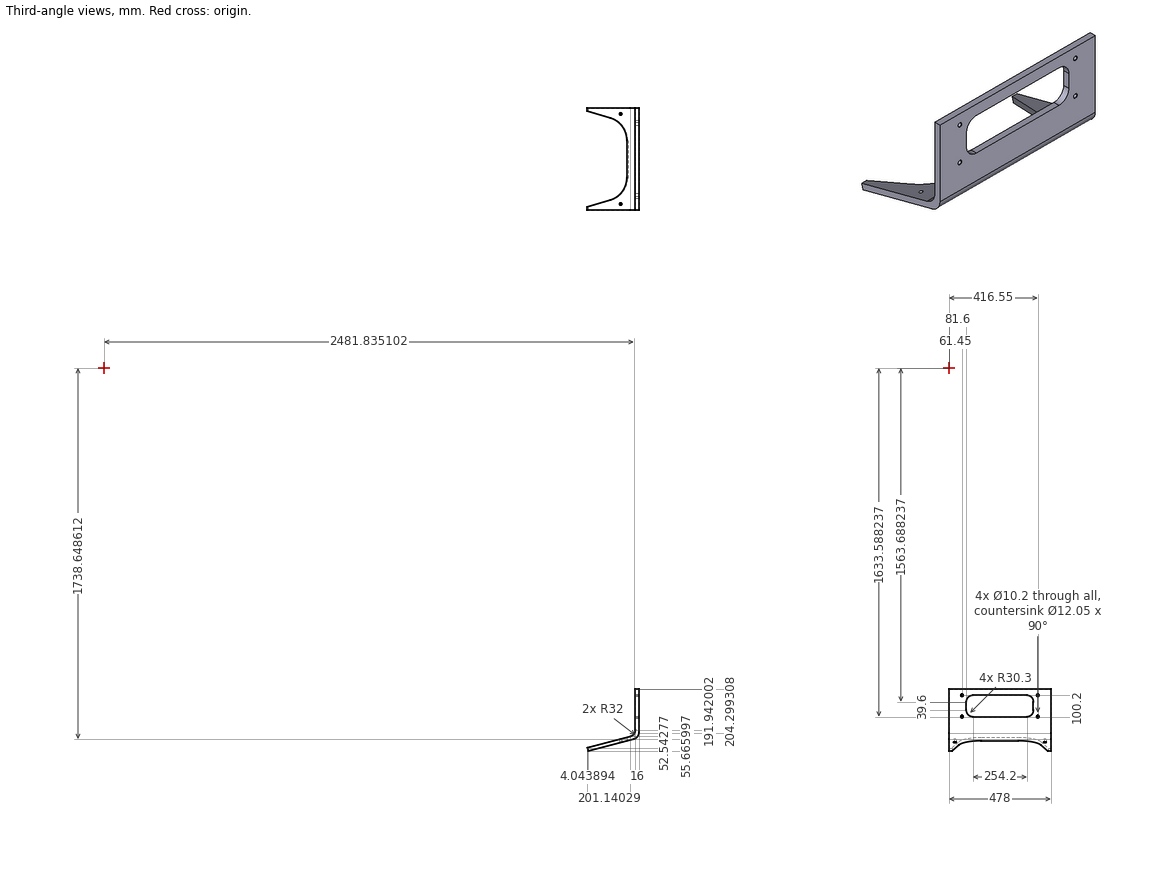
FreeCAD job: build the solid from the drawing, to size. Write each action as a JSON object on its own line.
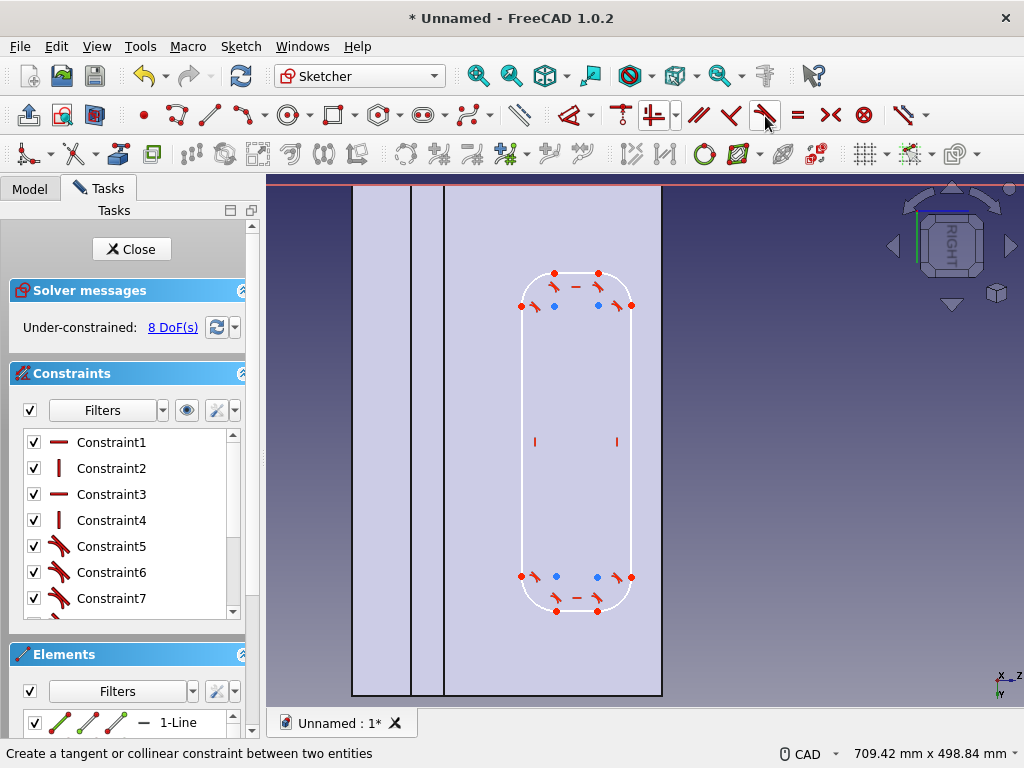
{"action": "left_click", "coordinate": [540, 277]}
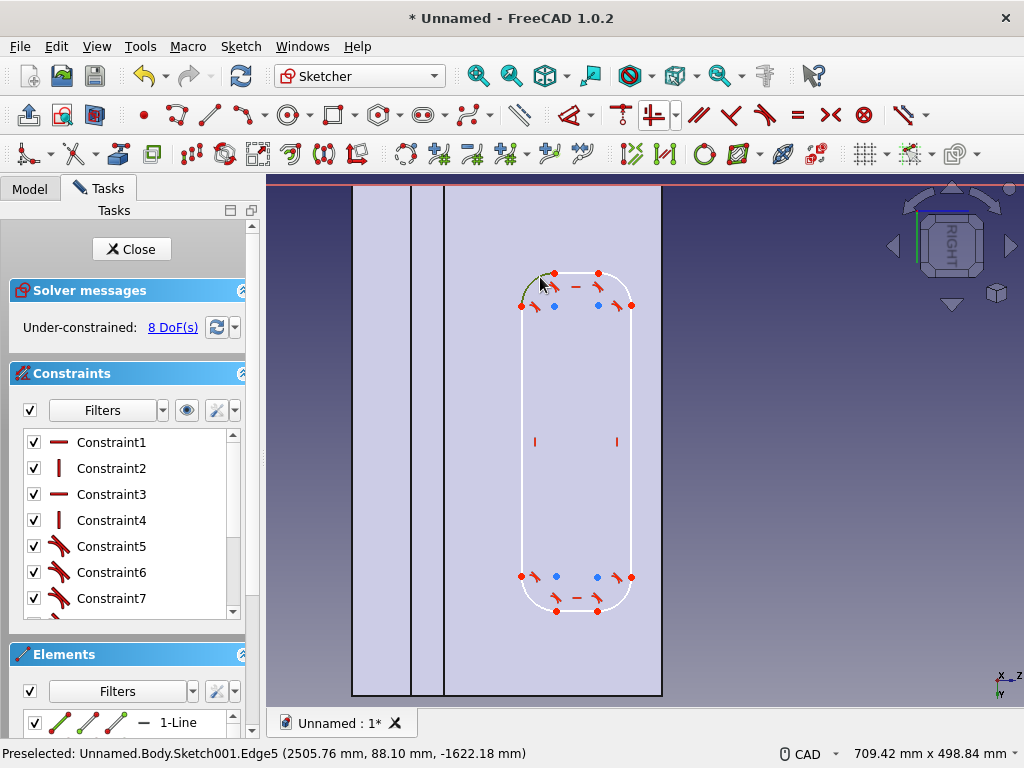
{"action": "left_click", "coordinate": [526, 592]}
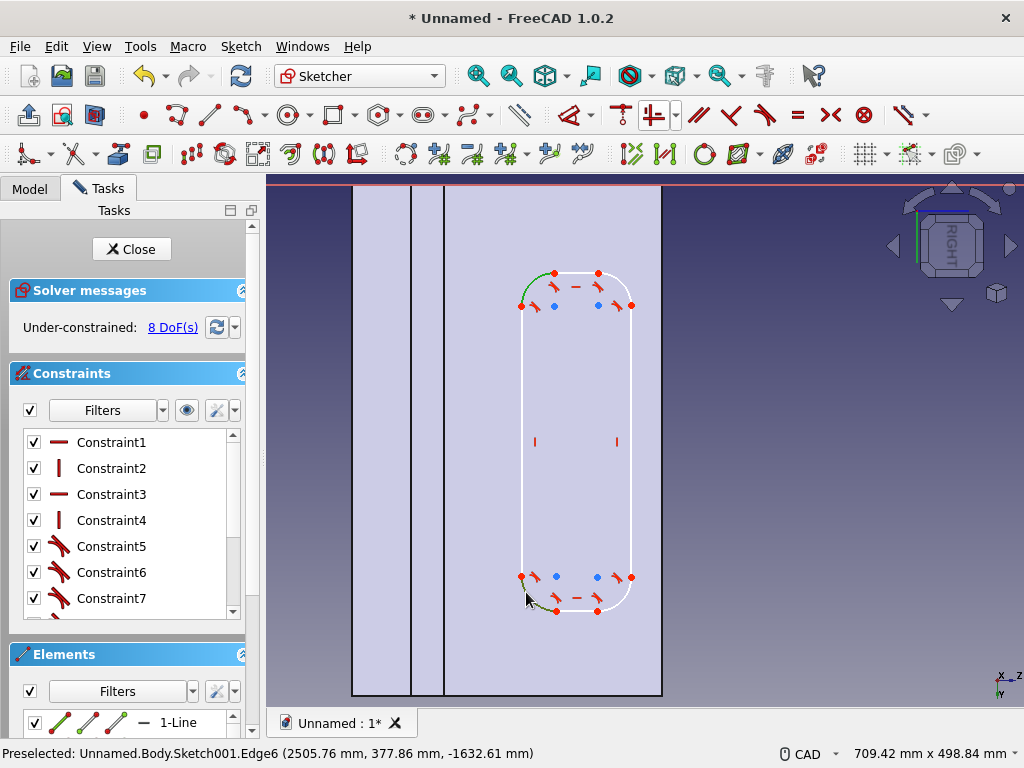
{"action": "left_click", "coordinate": [613, 607]}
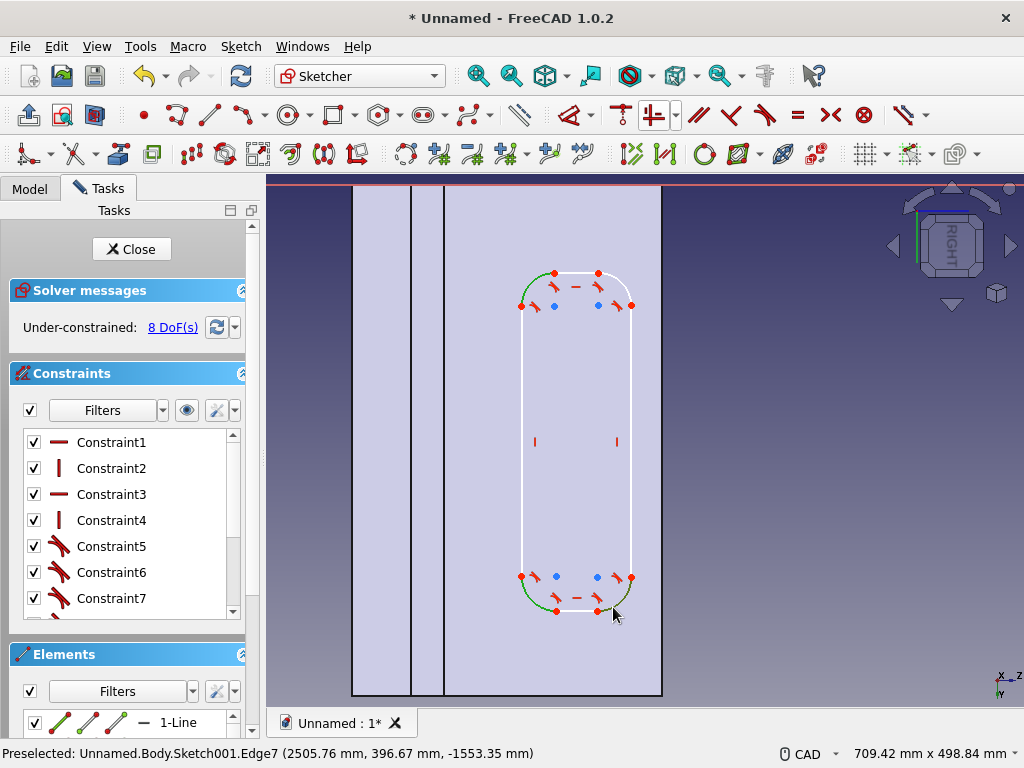
{"action": "left_click", "coordinate": [628, 291]}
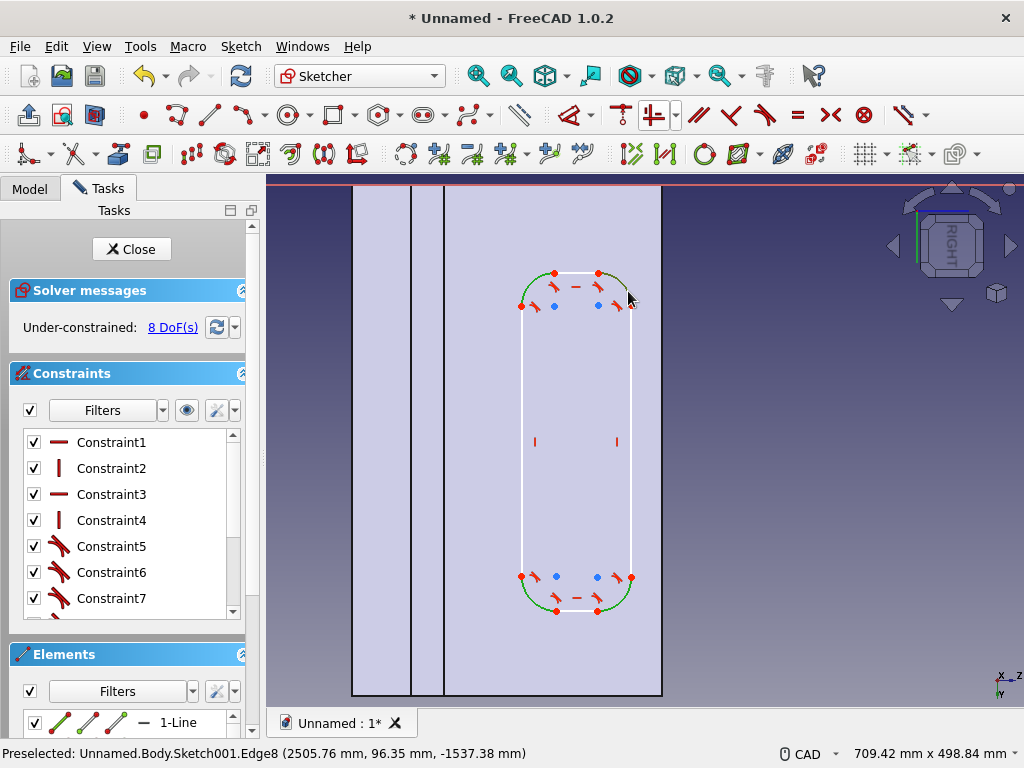
{"action": "left_click", "coordinate": [798, 116]}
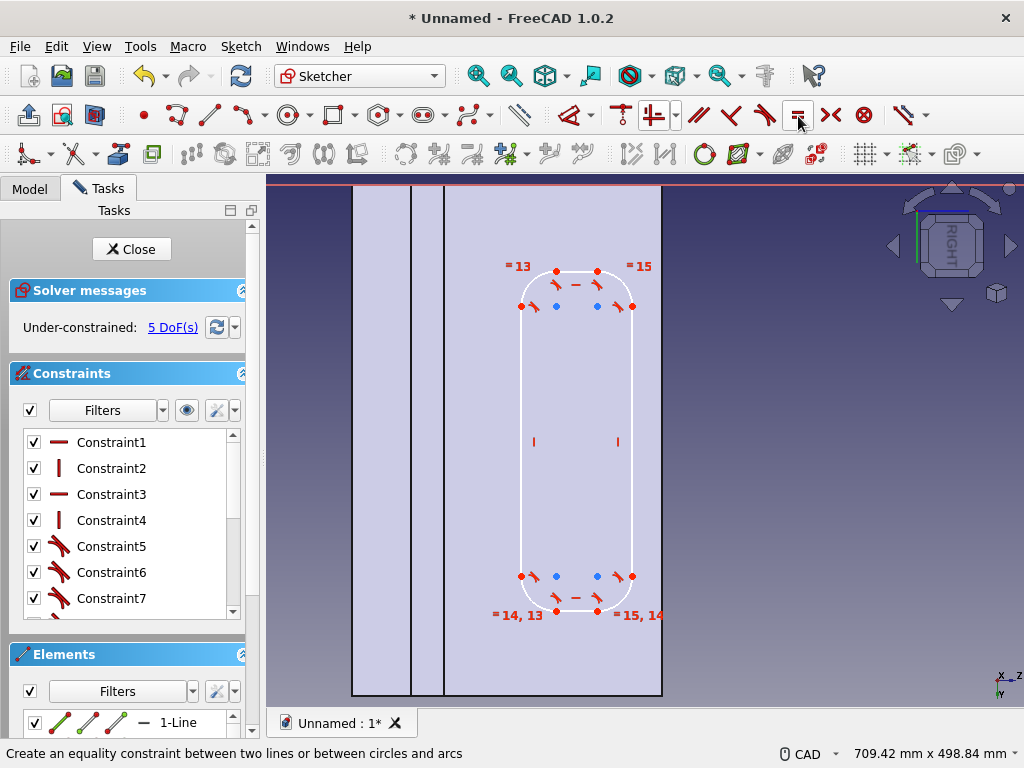
{"action": "left_click", "coordinate": [568, 116]}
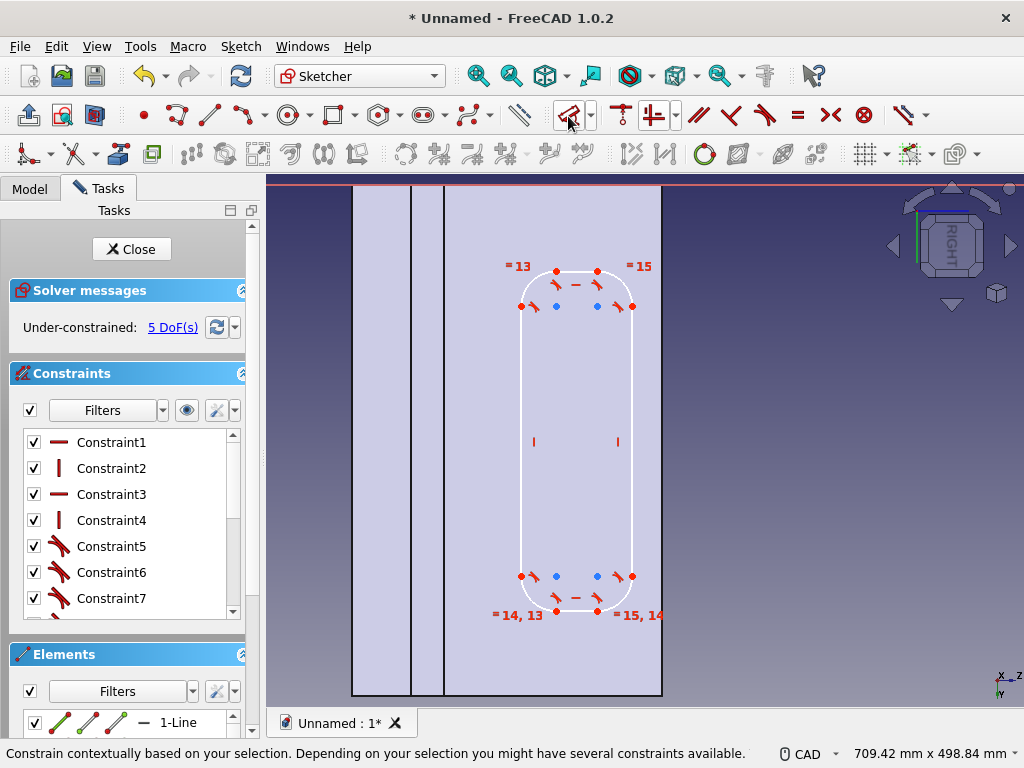
{"action": "scroll", "coordinate": [541, 275], "scroll_direction": "up", "scroll_amount": 2}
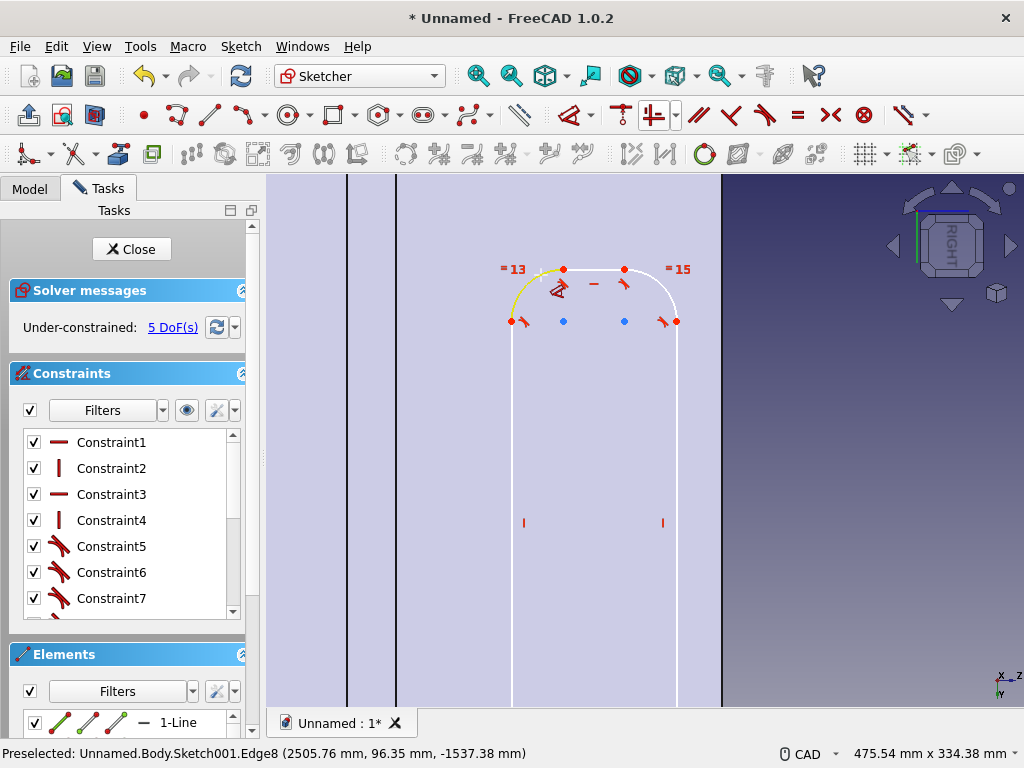
{"action": "left_click", "coordinate": [540, 275]}
{"action": "left_click", "coordinate": [526, 246]}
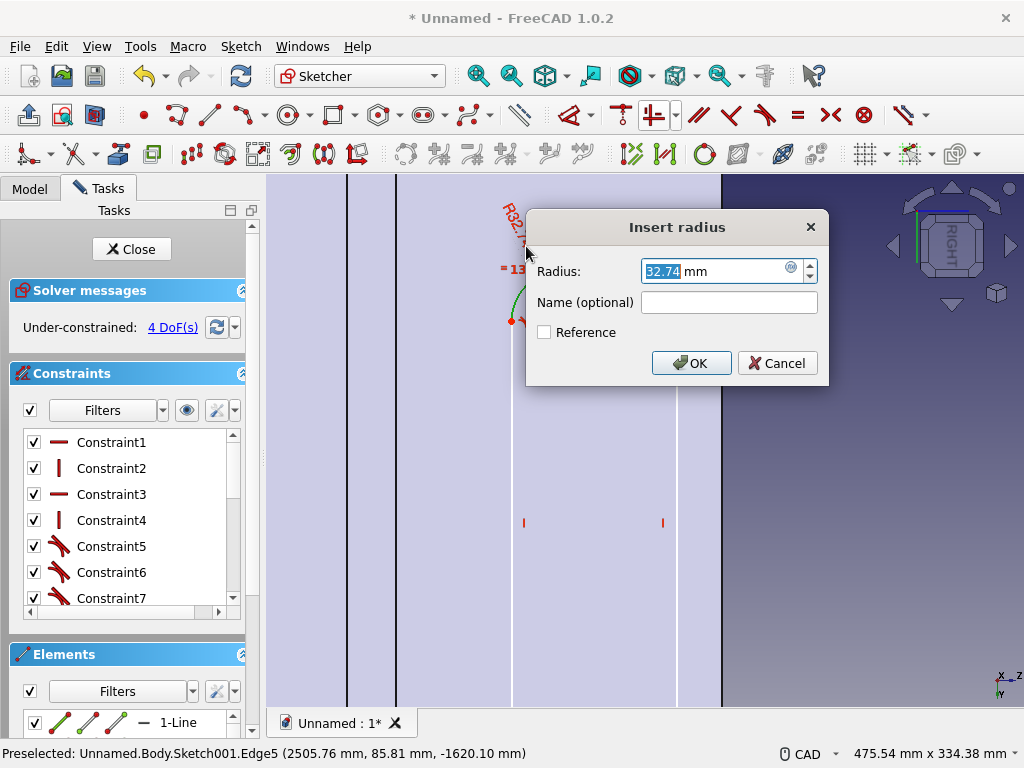
{"action": "type", "text": "30.3"}
{"action": "key", "text": "Return"}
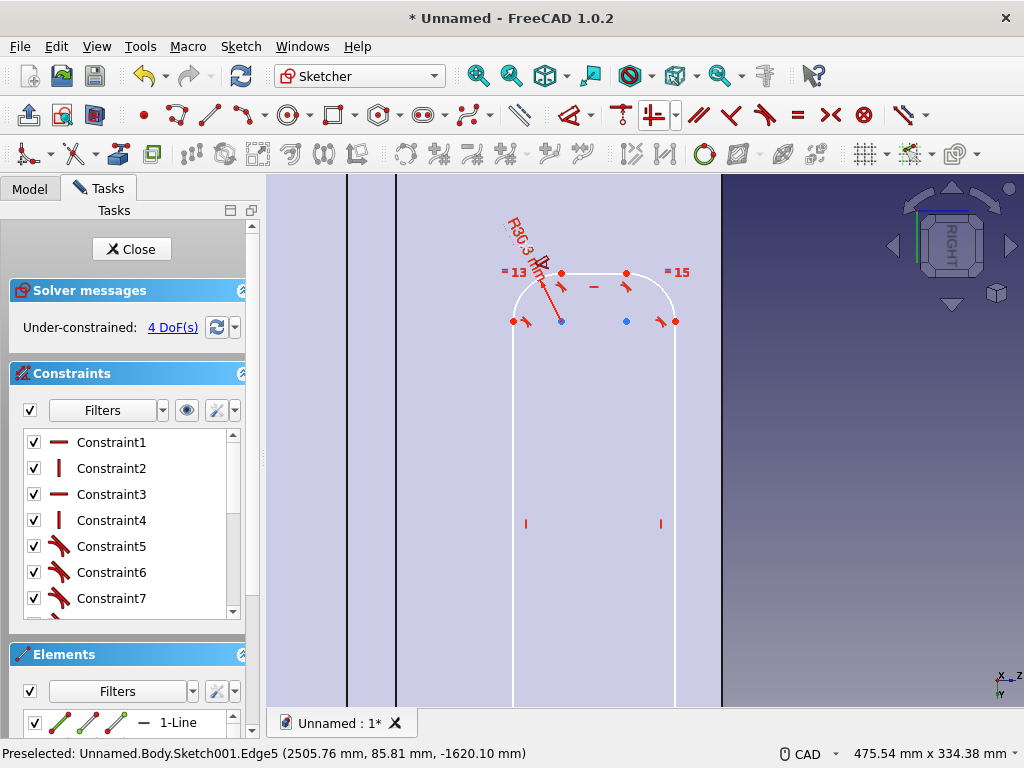
{"action": "left_click", "coordinate": [607, 274]}
{"action": "left_click", "coordinate": [609, 240]}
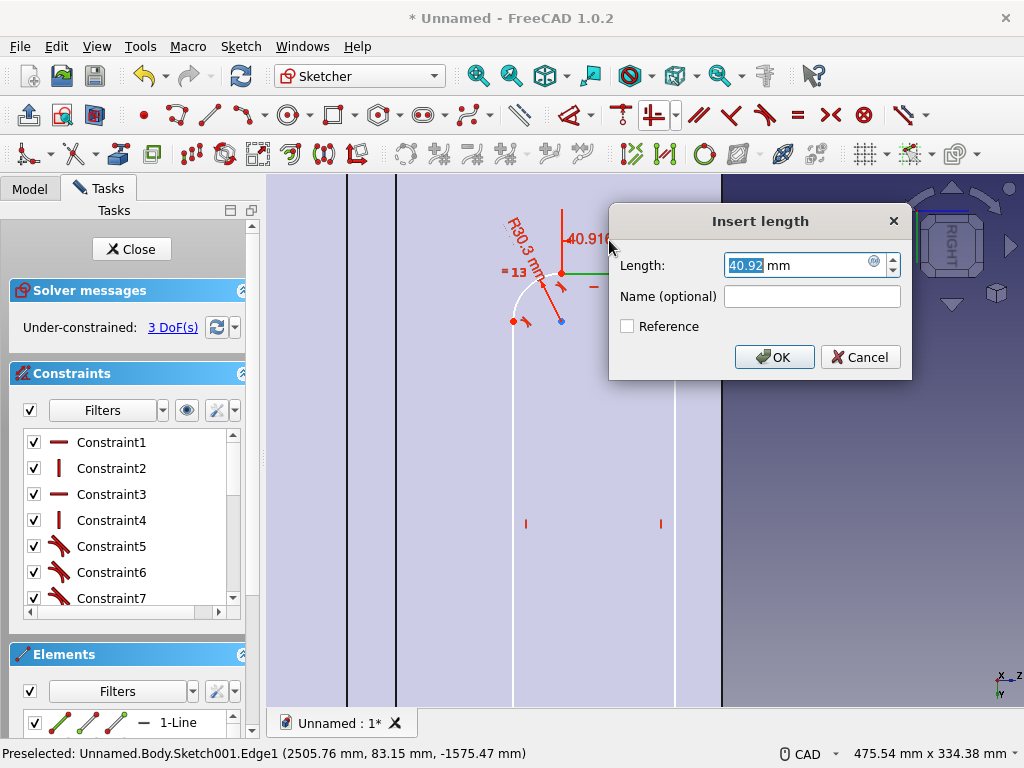
{"action": "type", "text": "39.6"}
{"action": "key", "text": "Return"}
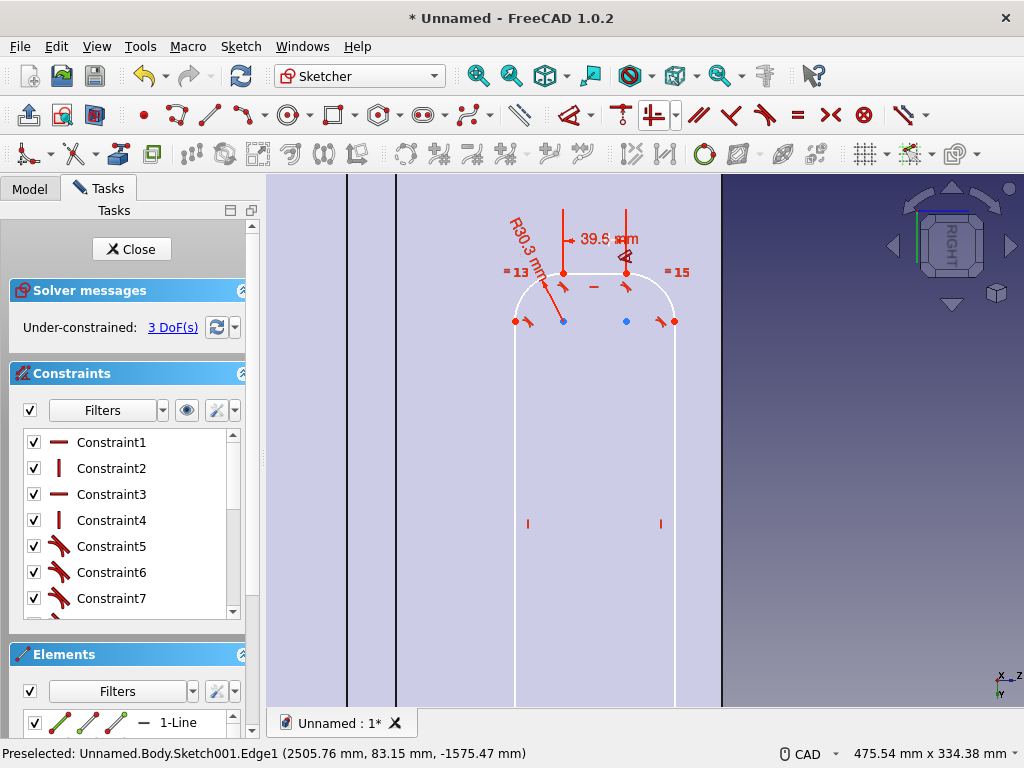
{"action": "left_click", "coordinate": [515, 443]}
{"action": "left_click", "coordinate": [481, 500]}